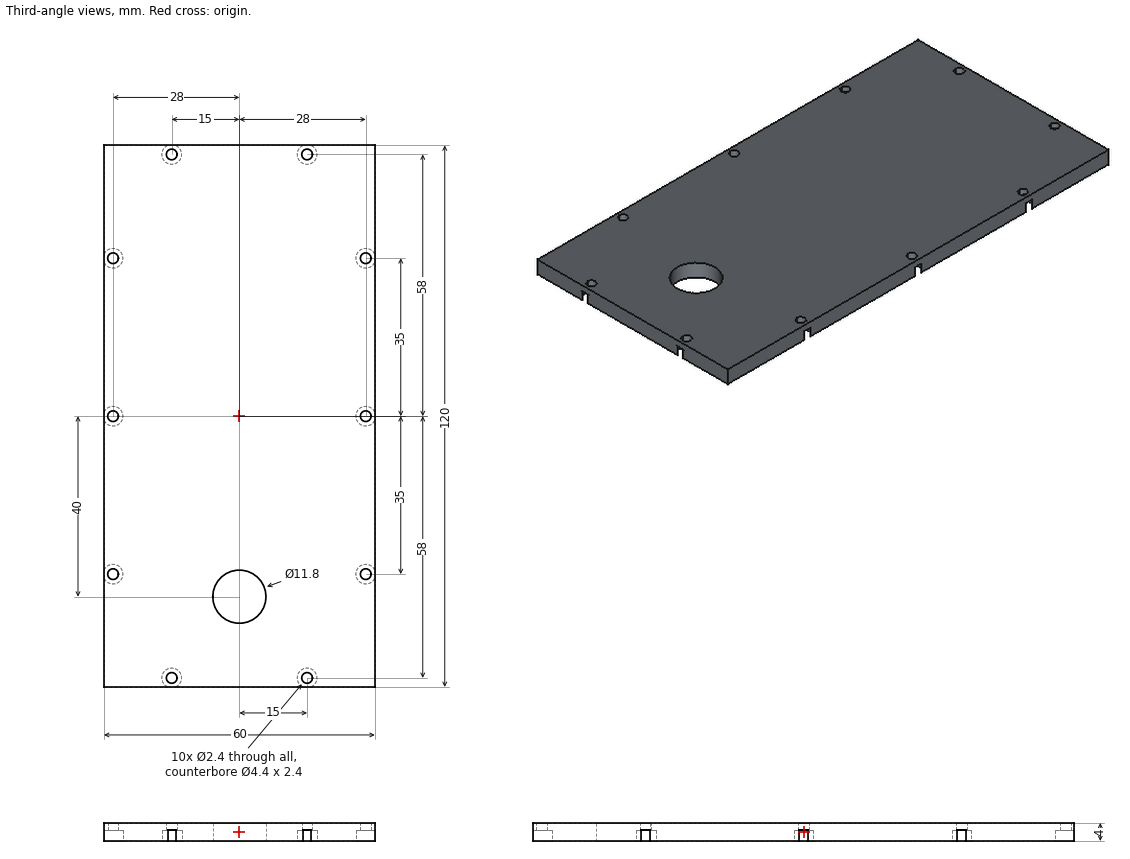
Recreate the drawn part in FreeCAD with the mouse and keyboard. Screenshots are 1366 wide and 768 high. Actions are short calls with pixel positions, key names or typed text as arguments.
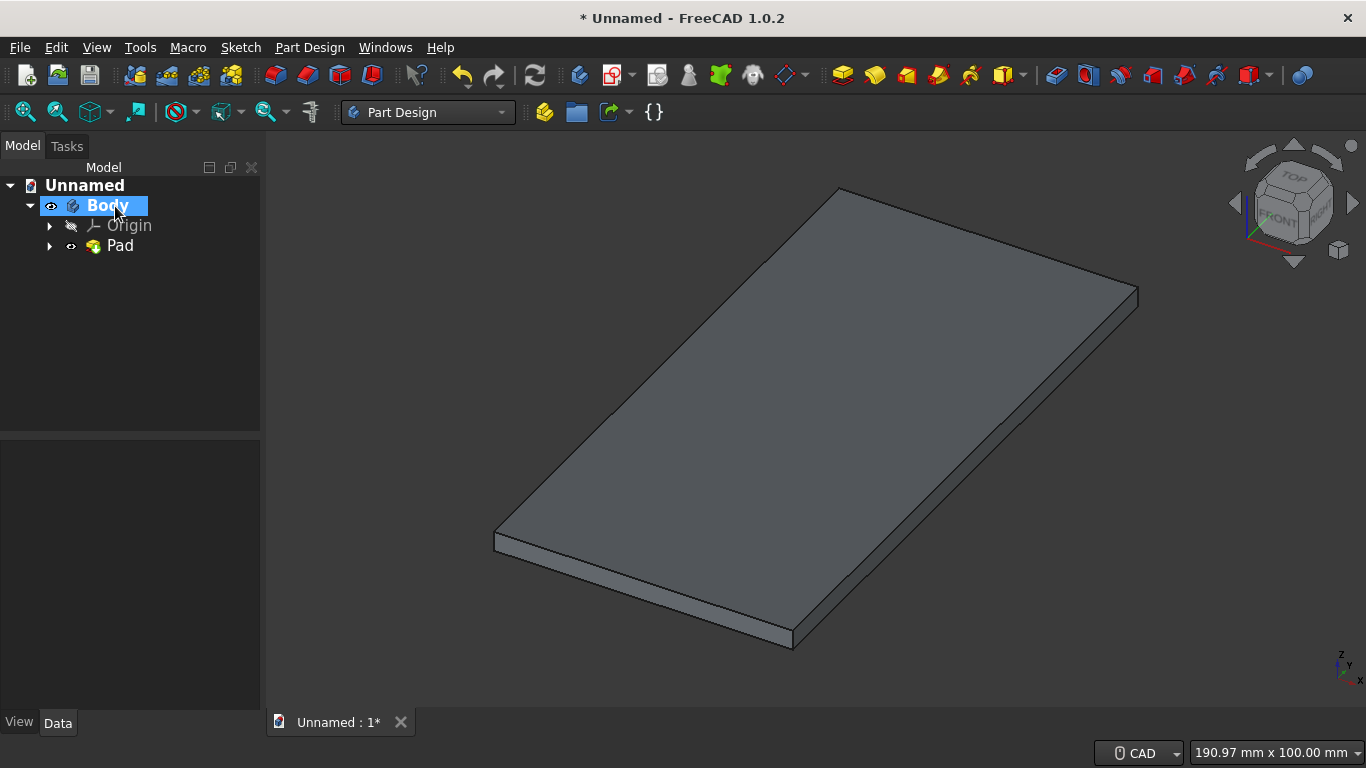
key(5)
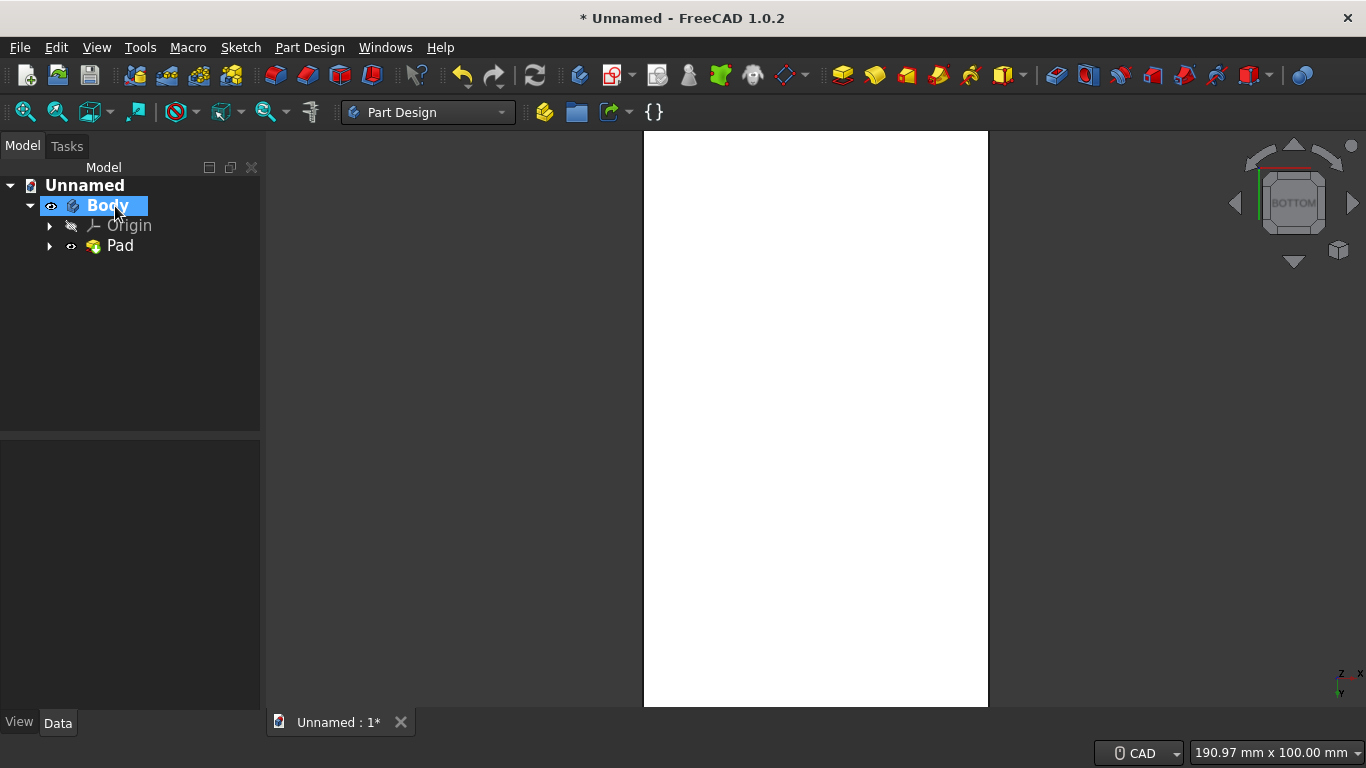
click(26, 112)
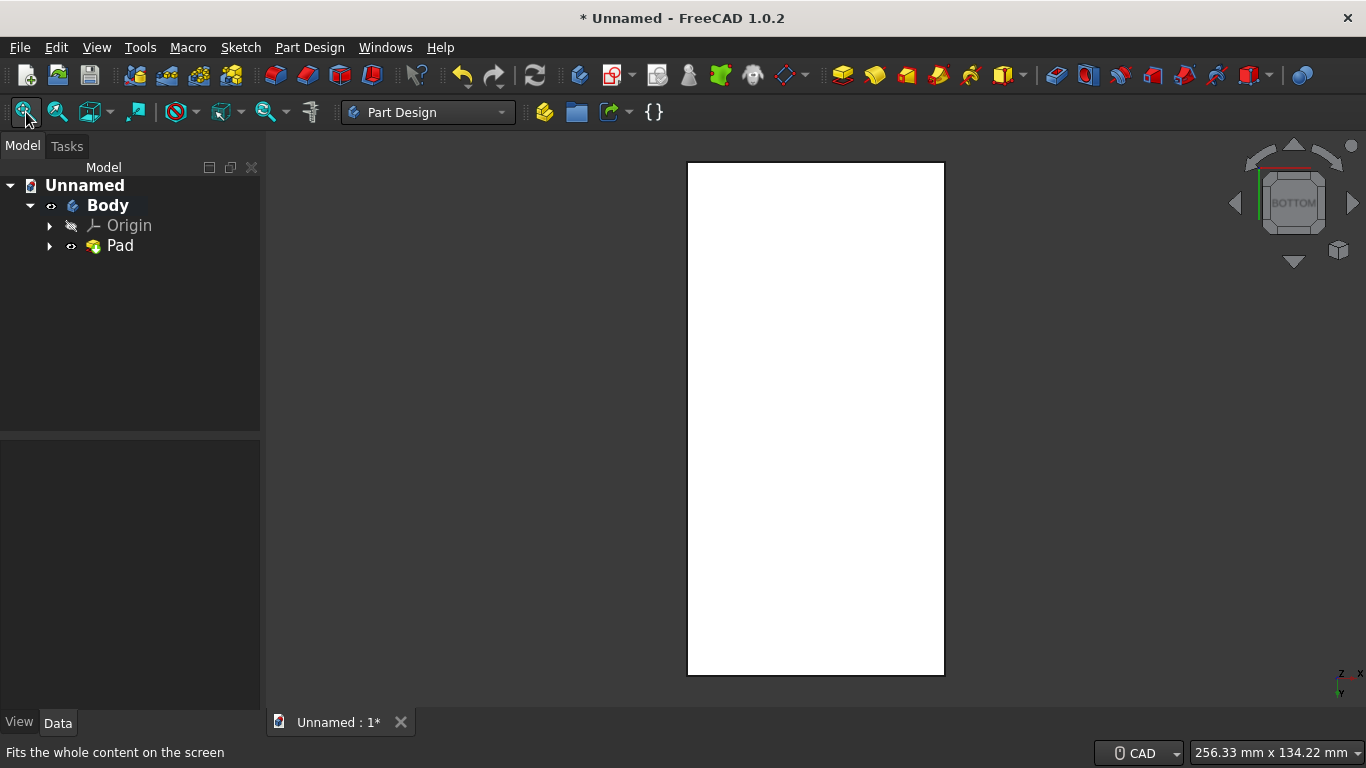
click(816, 492)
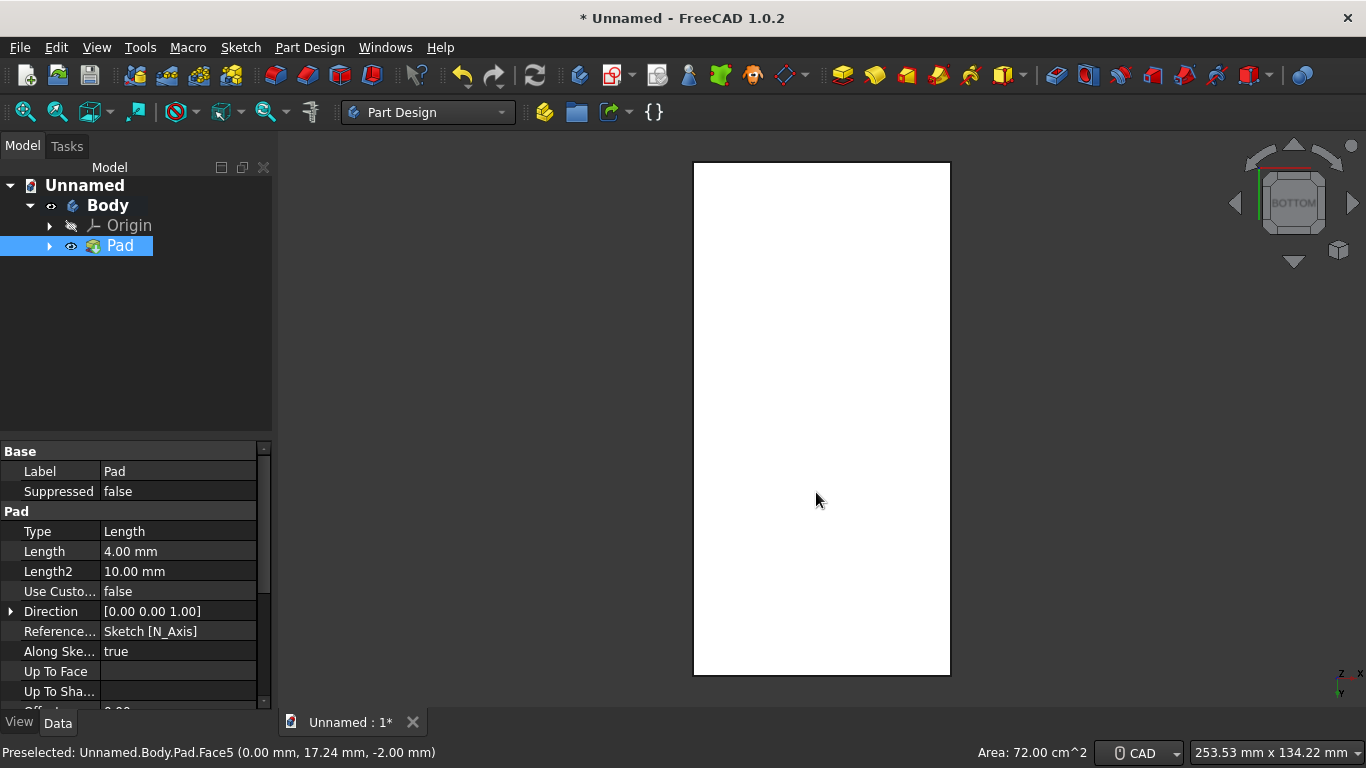
click(612, 76)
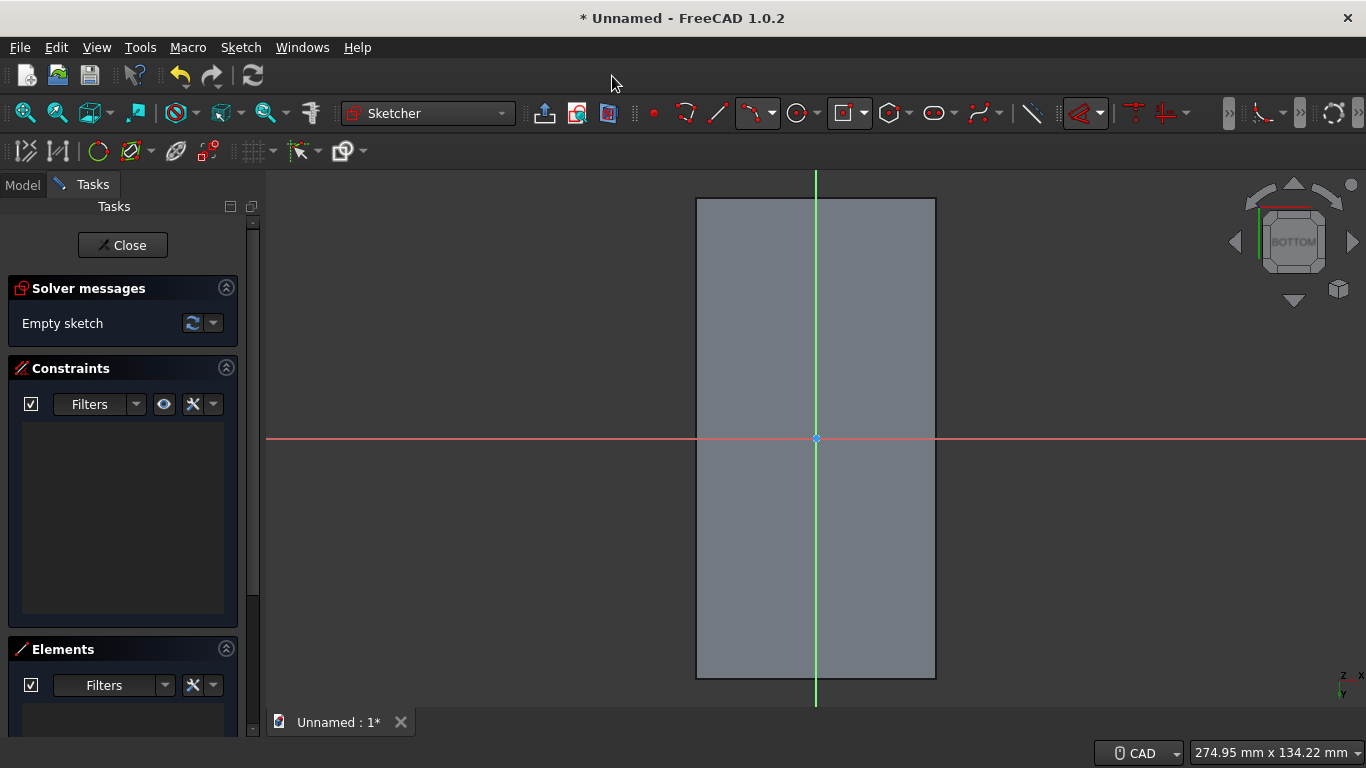
scroll(608, 438, down, 2)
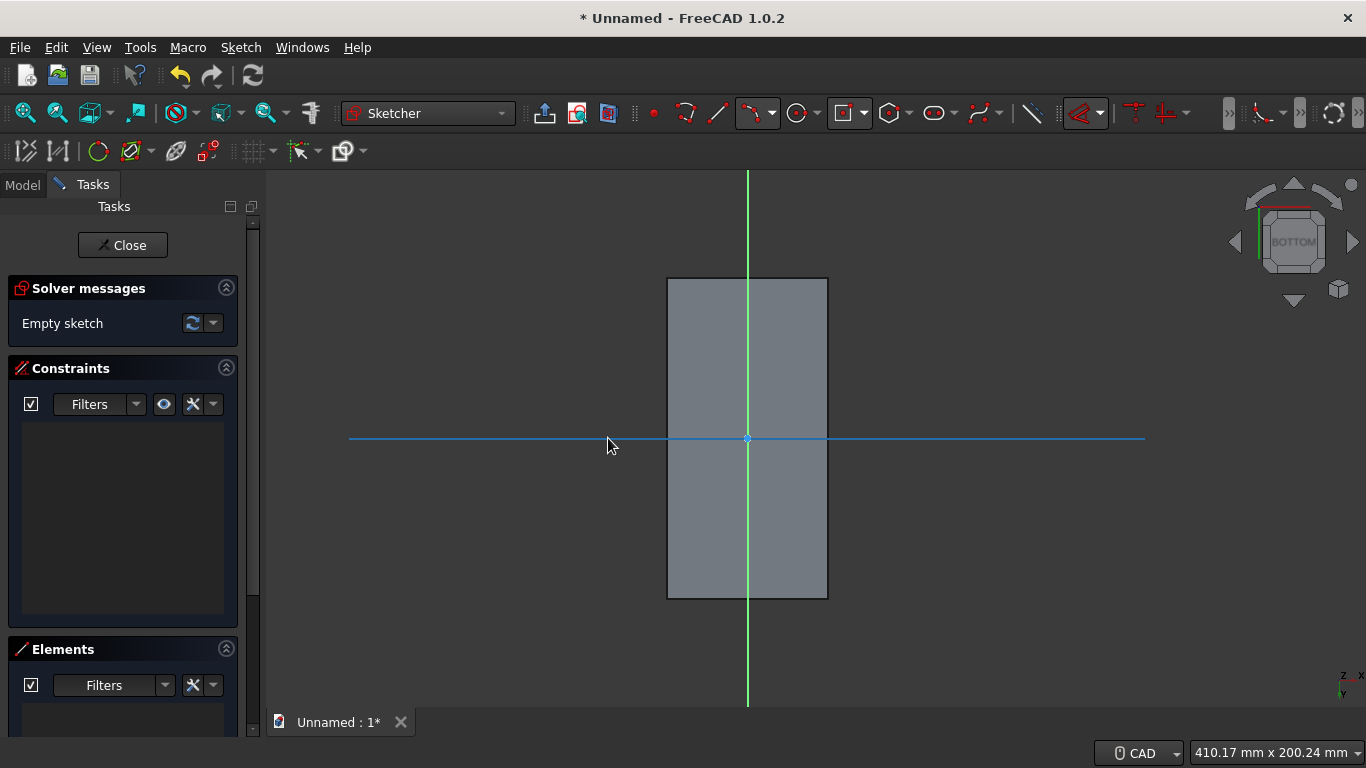
click(798, 114)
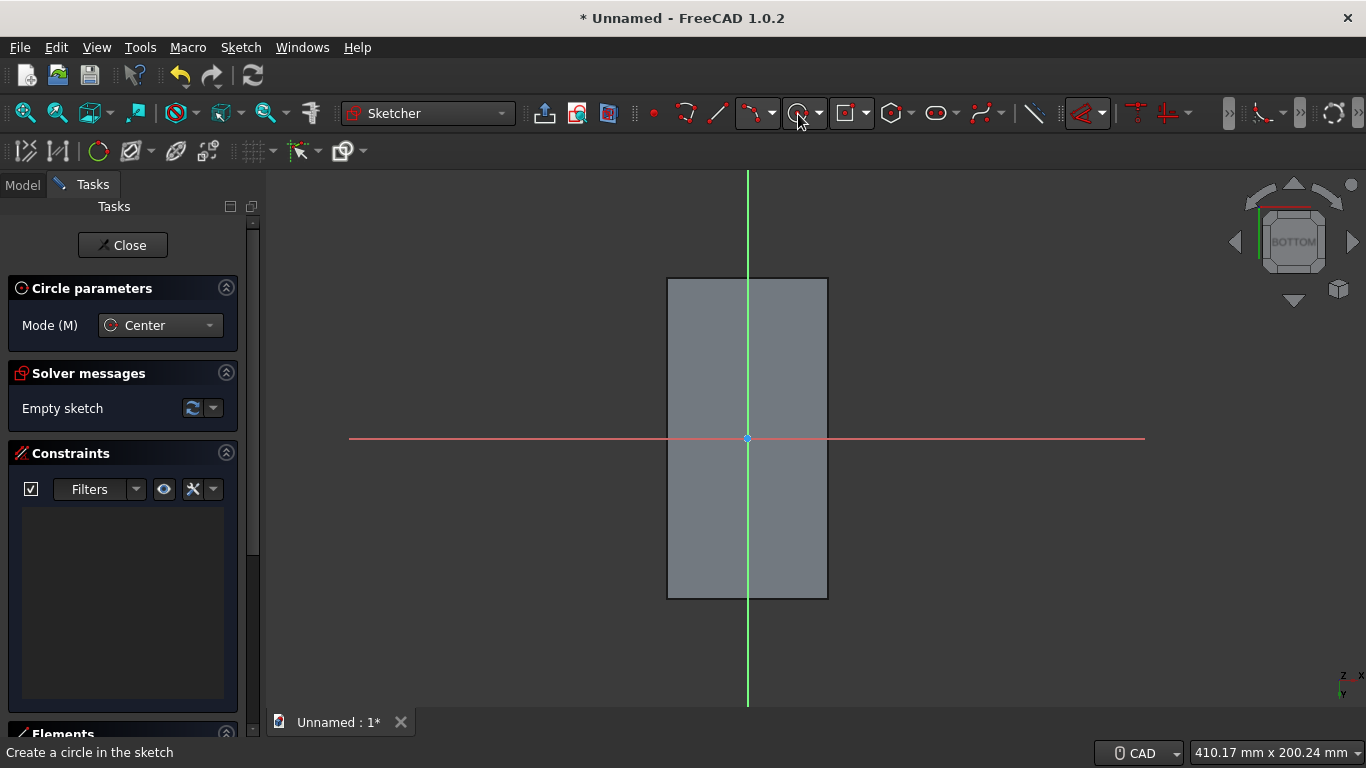
scroll(788, 283, up, 10)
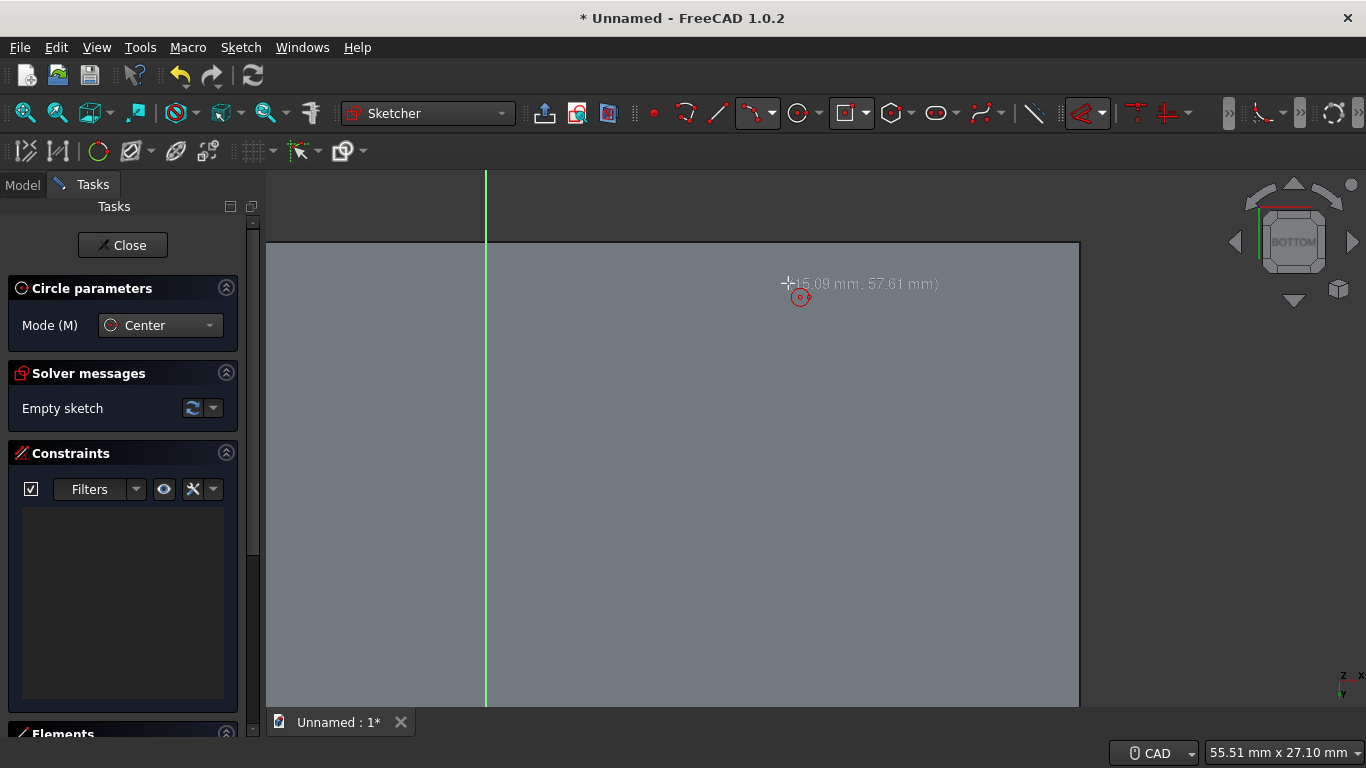
scroll(788, 283, down, 10)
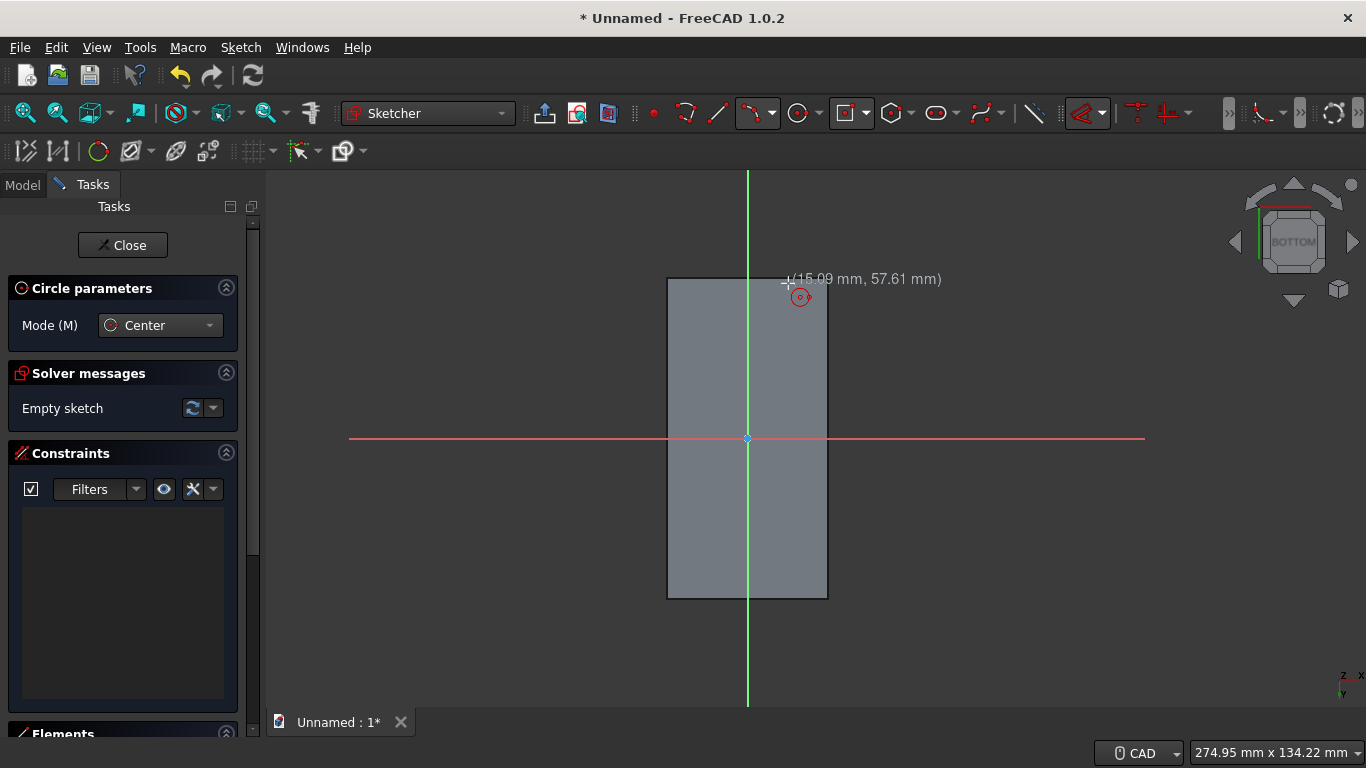
click(788, 283)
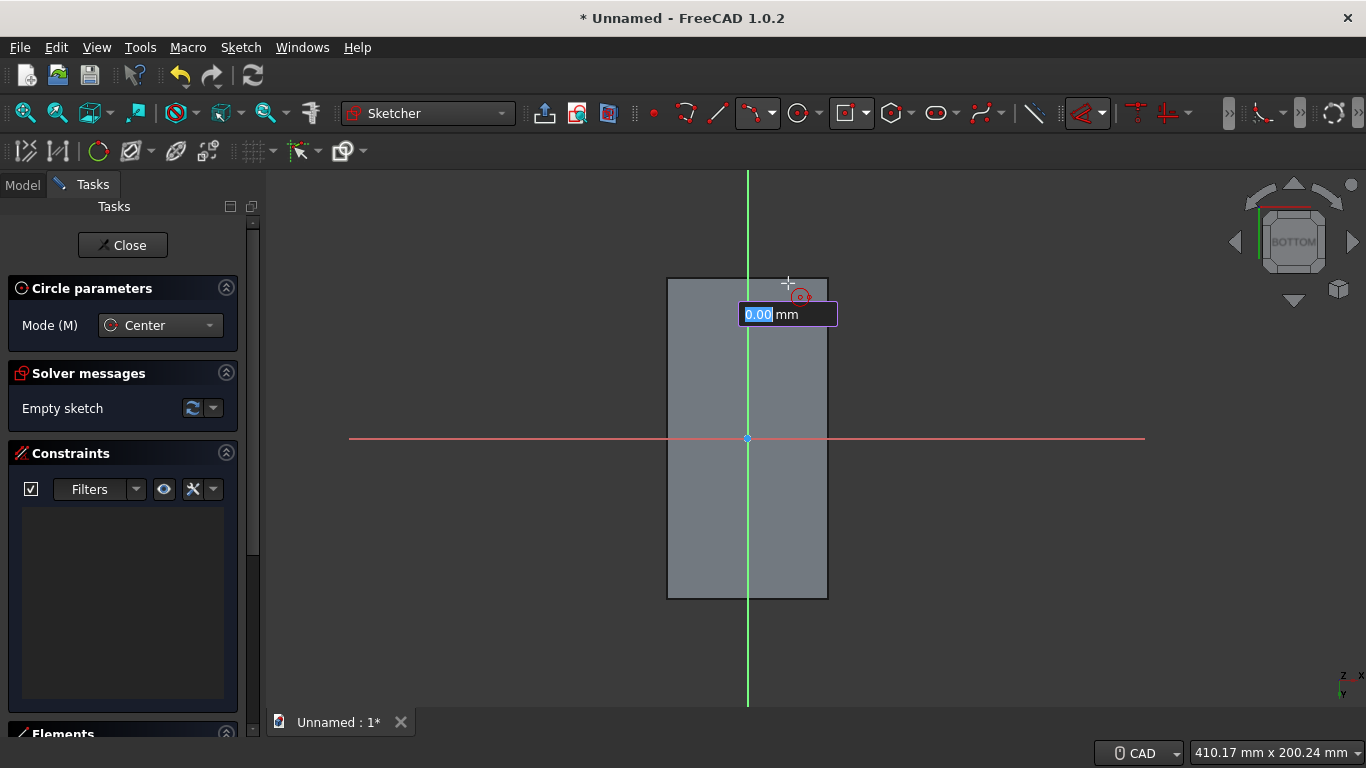
scroll(790, 281, up, 8)